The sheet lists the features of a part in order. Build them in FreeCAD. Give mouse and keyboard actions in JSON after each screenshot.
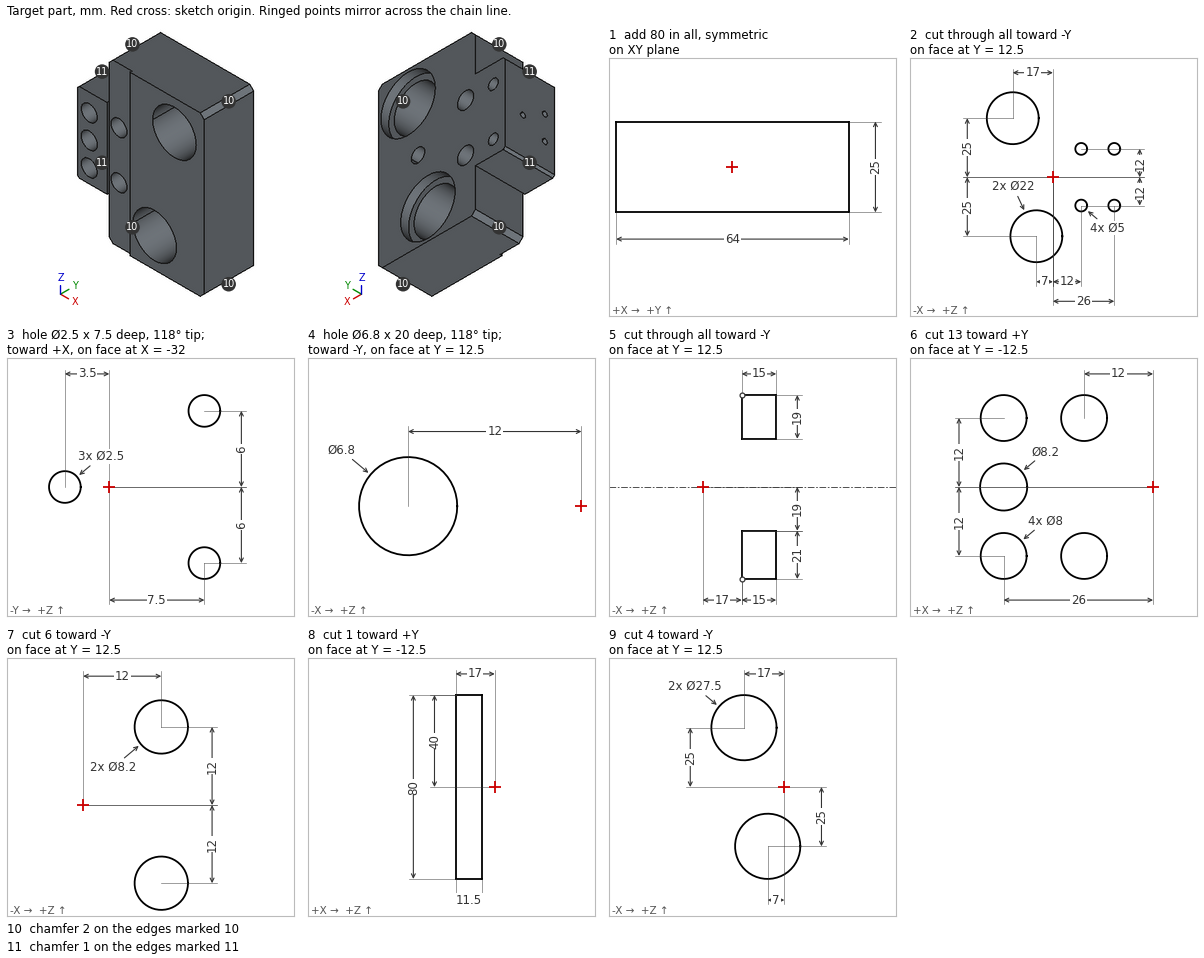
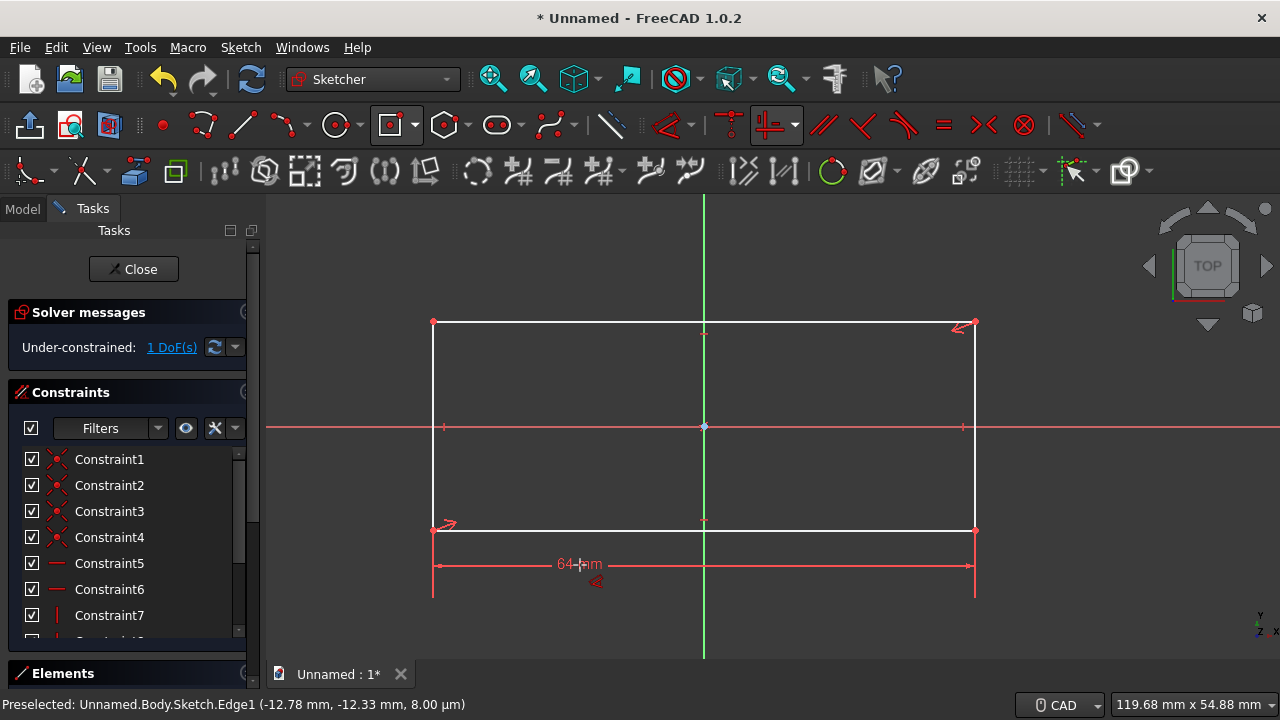
{"action": "left_click", "coordinate": [975, 468]}
{"action": "left_click", "coordinate": [1009, 378]}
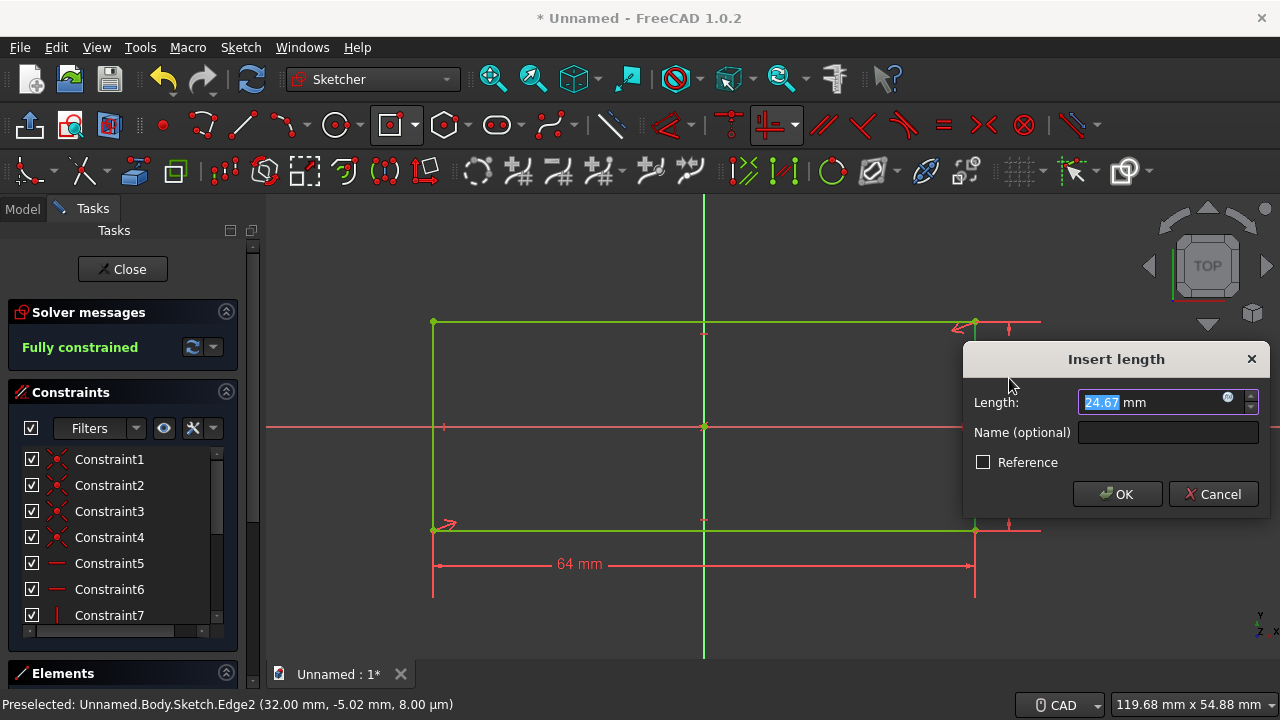
{"action": "type", "text": "25"}
{"action": "key", "text": "Return"}
{"action": "key", "text": "Escape"}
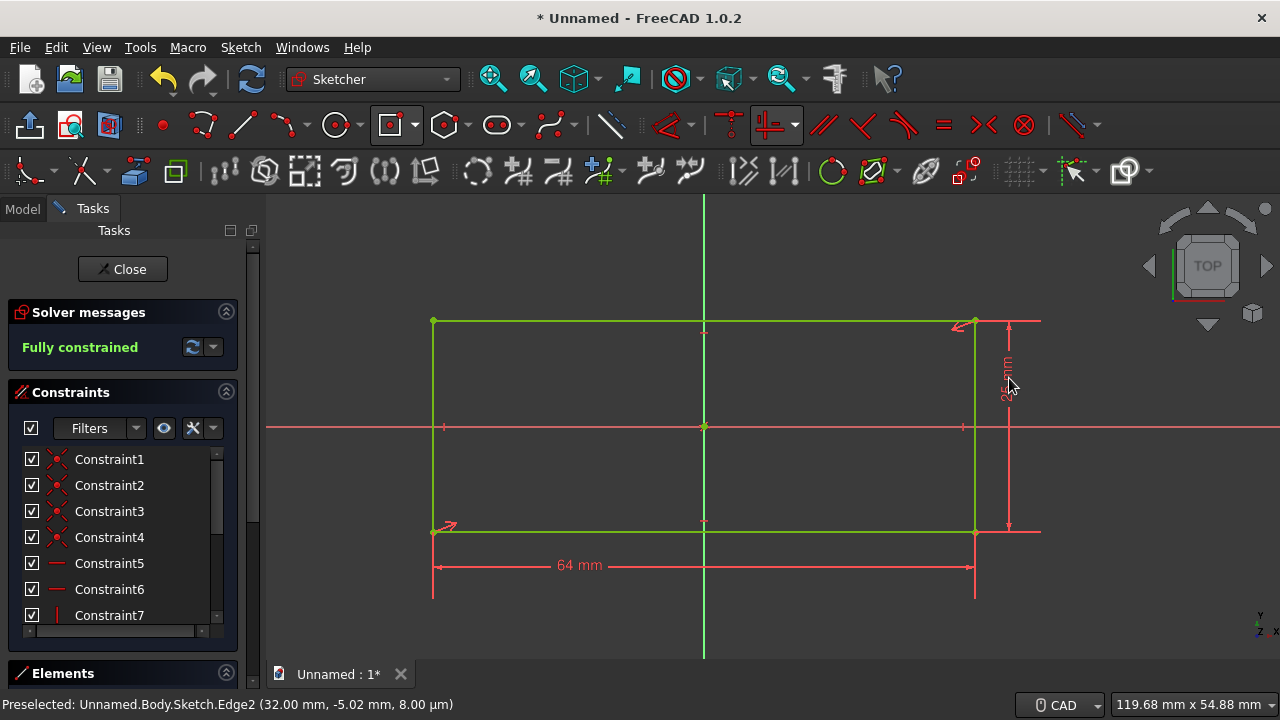
{"action": "left_click", "coordinate": [123, 269]}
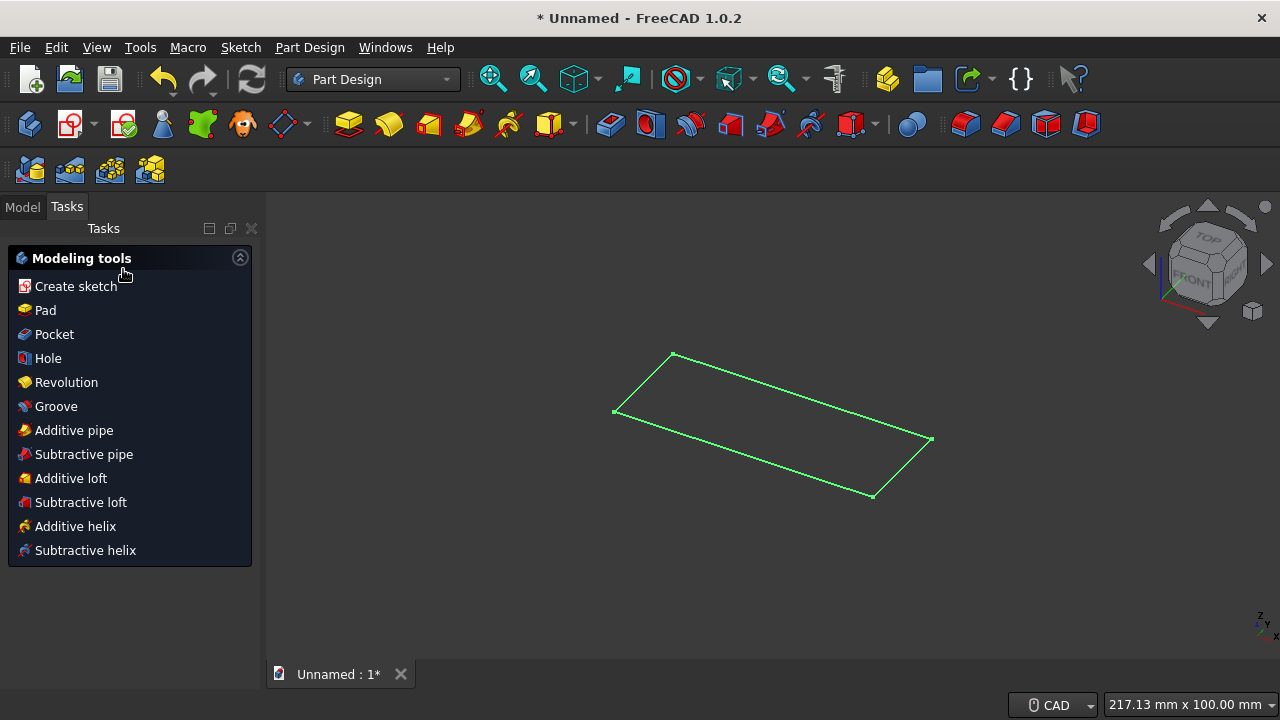
{"action": "left_click", "coordinate": [350, 124]}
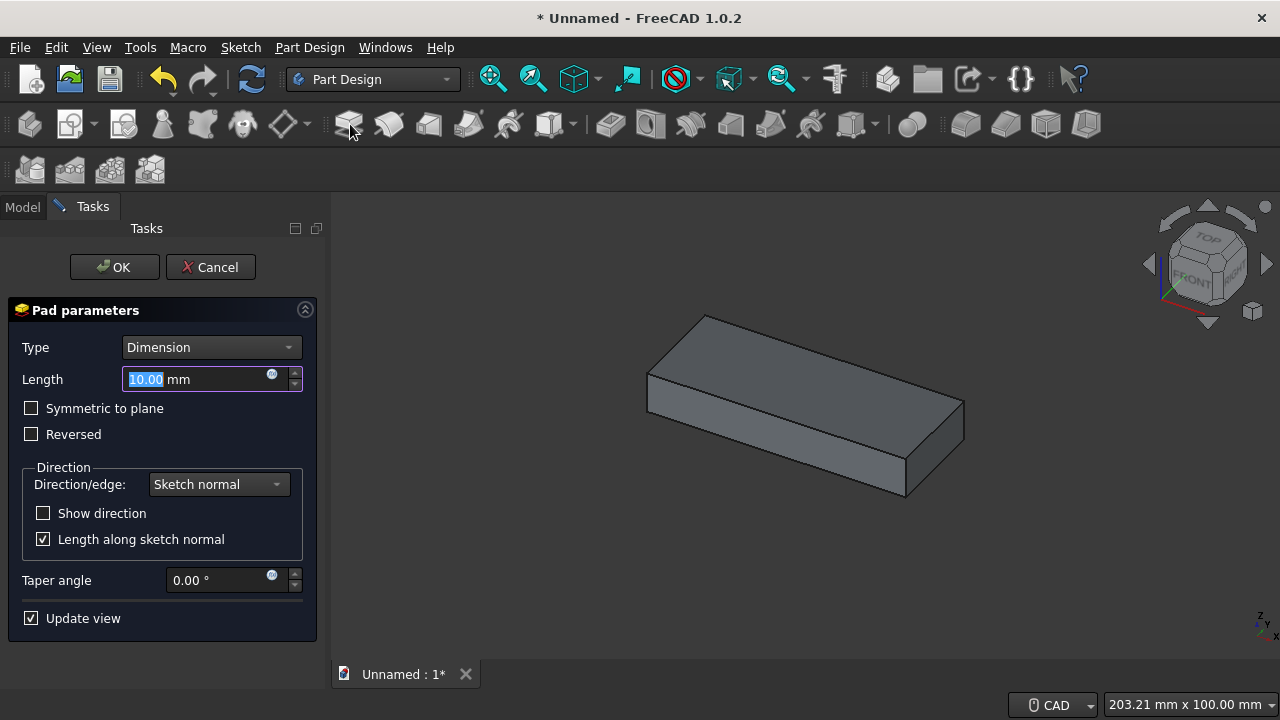
{"action": "type", "text": "80"}
{"action": "key", "text": "Tab"}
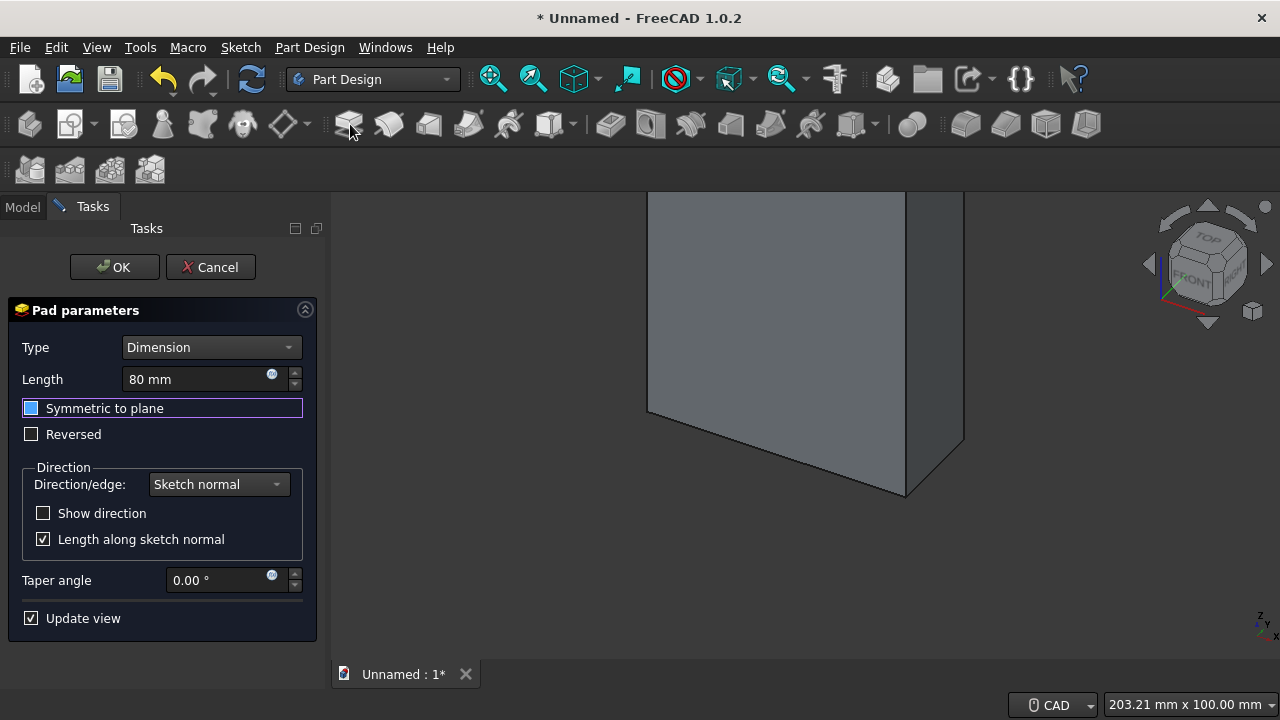
{"action": "left_click", "coordinate": [30, 408]}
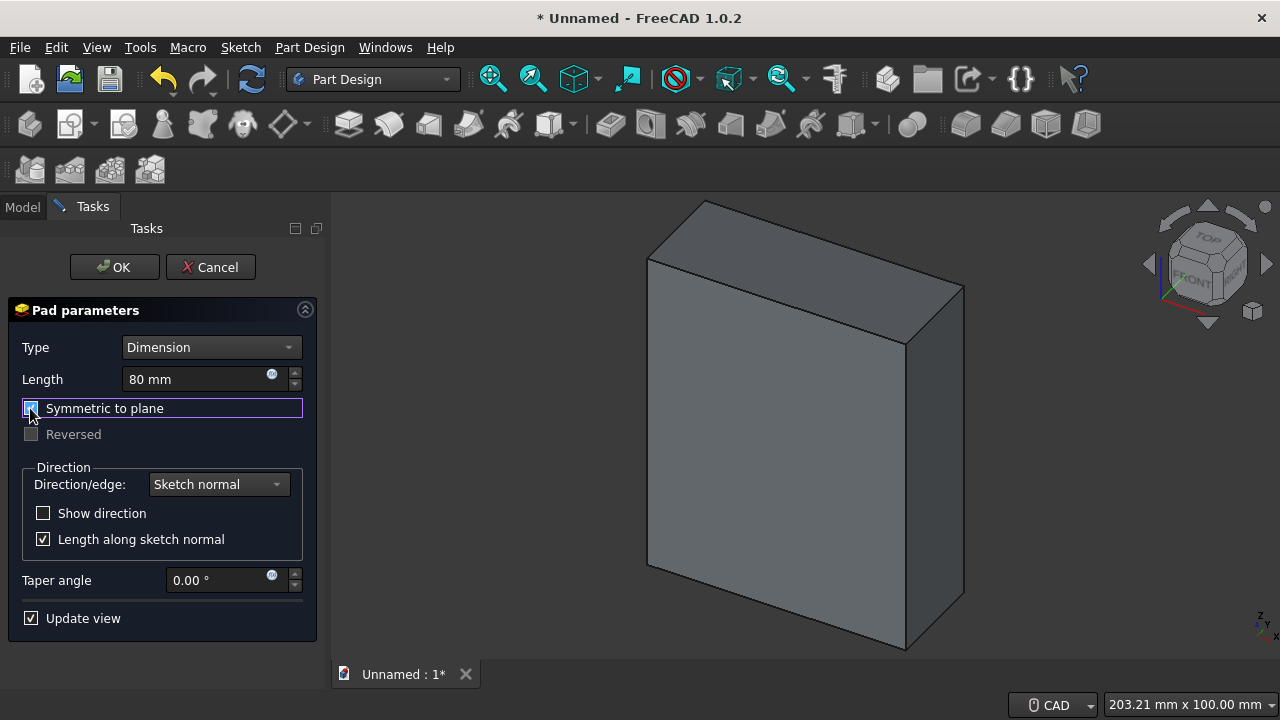
{"action": "left_click", "coordinate": [115, 267]}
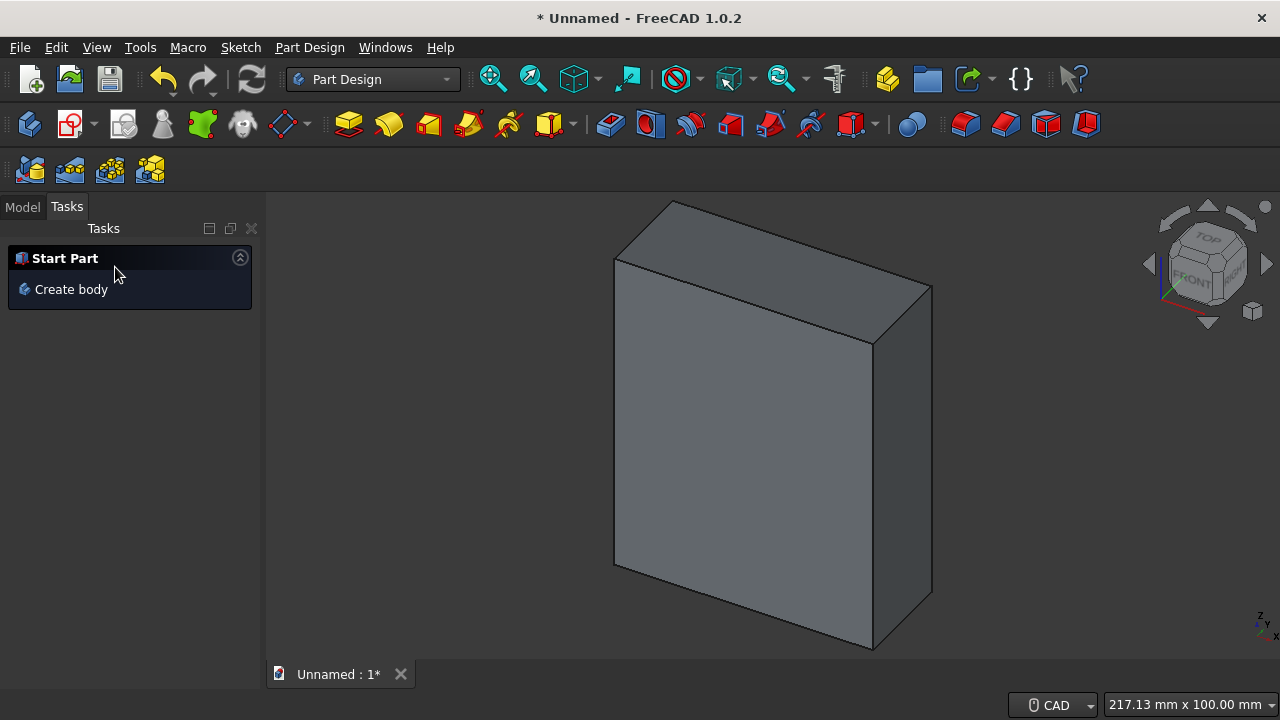
{"action": "key", "text": "4"}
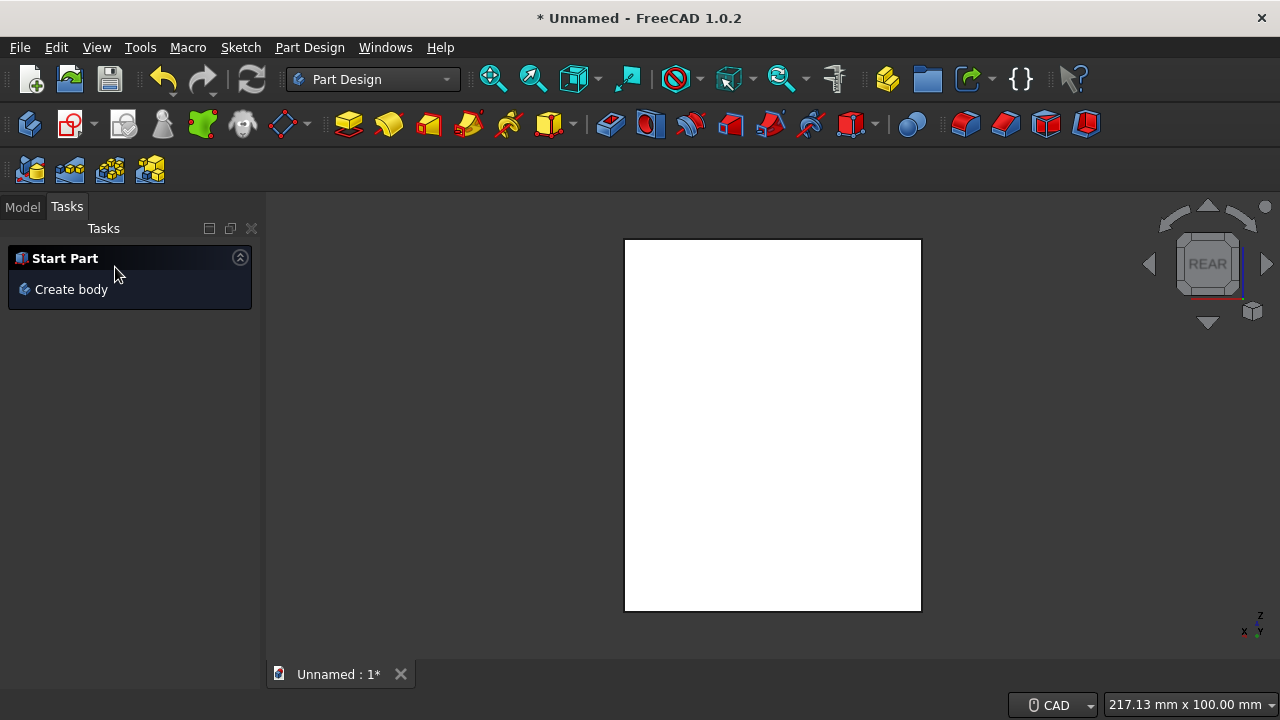
{"action": "left_click", "coordinate": [773, 424]}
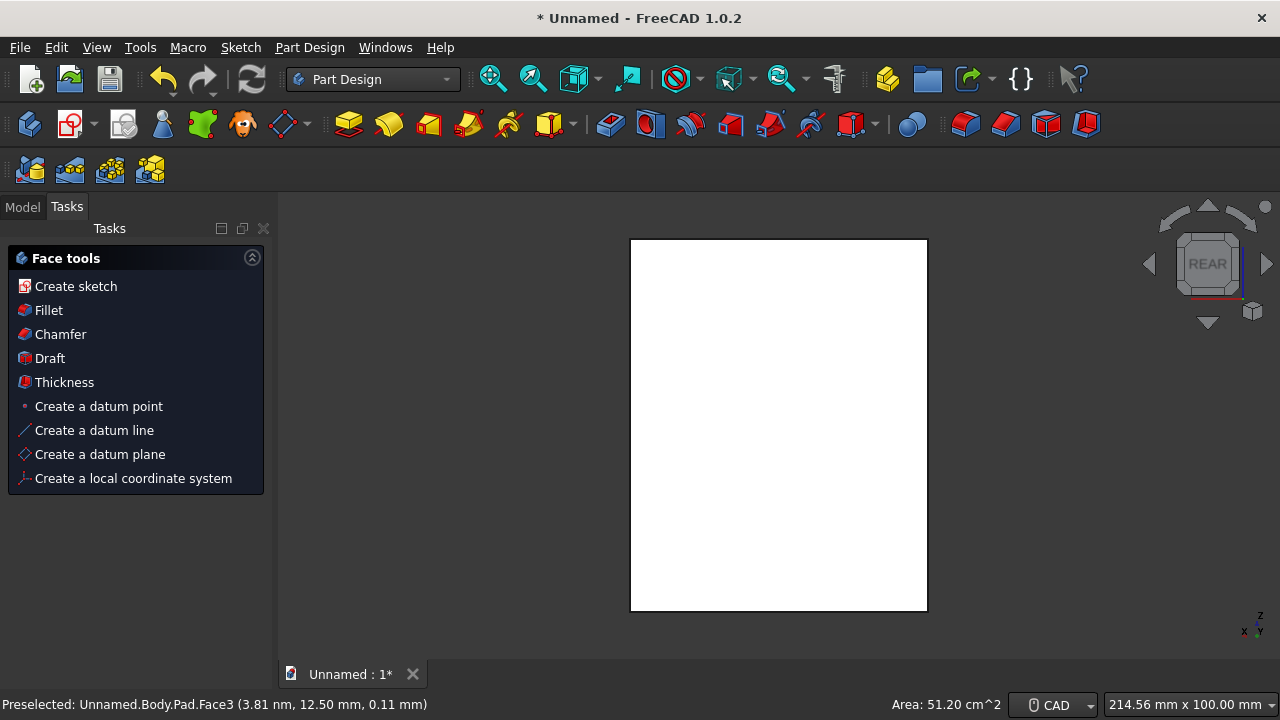
{"action": "left_click", "coordinate": [70, 124]}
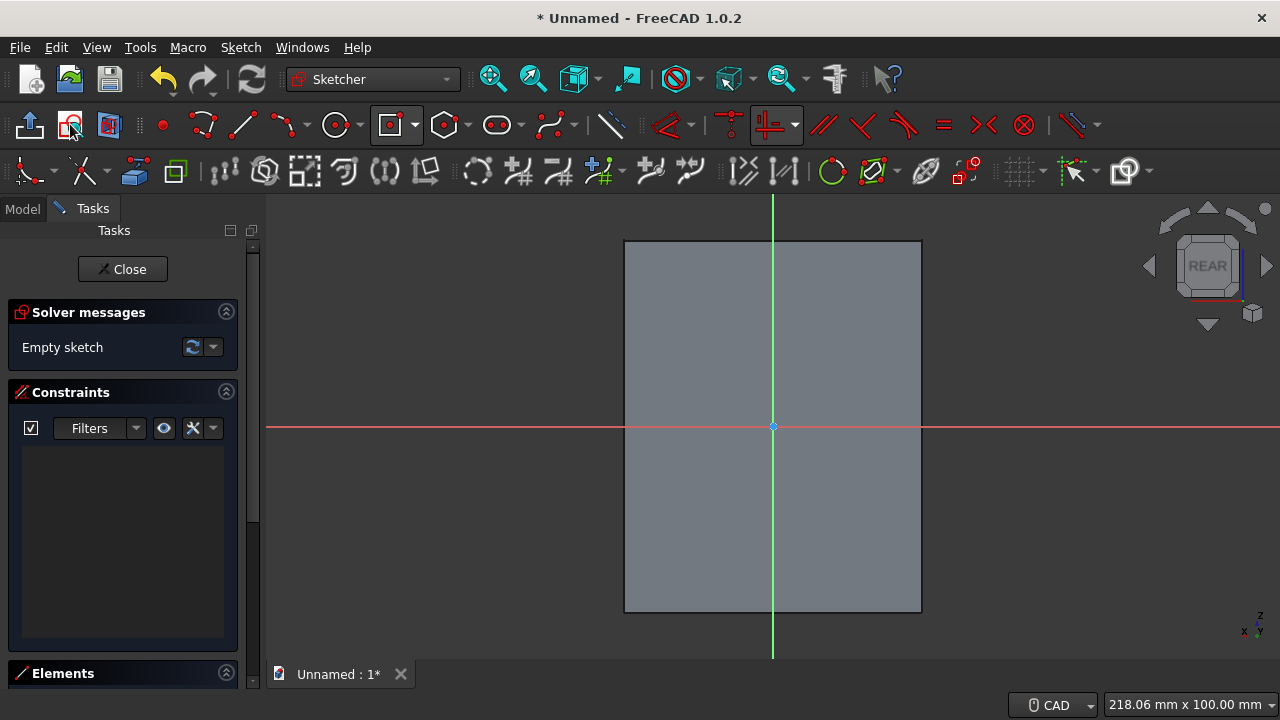
{"action": "left_click", "coordinate": [336, 126]}